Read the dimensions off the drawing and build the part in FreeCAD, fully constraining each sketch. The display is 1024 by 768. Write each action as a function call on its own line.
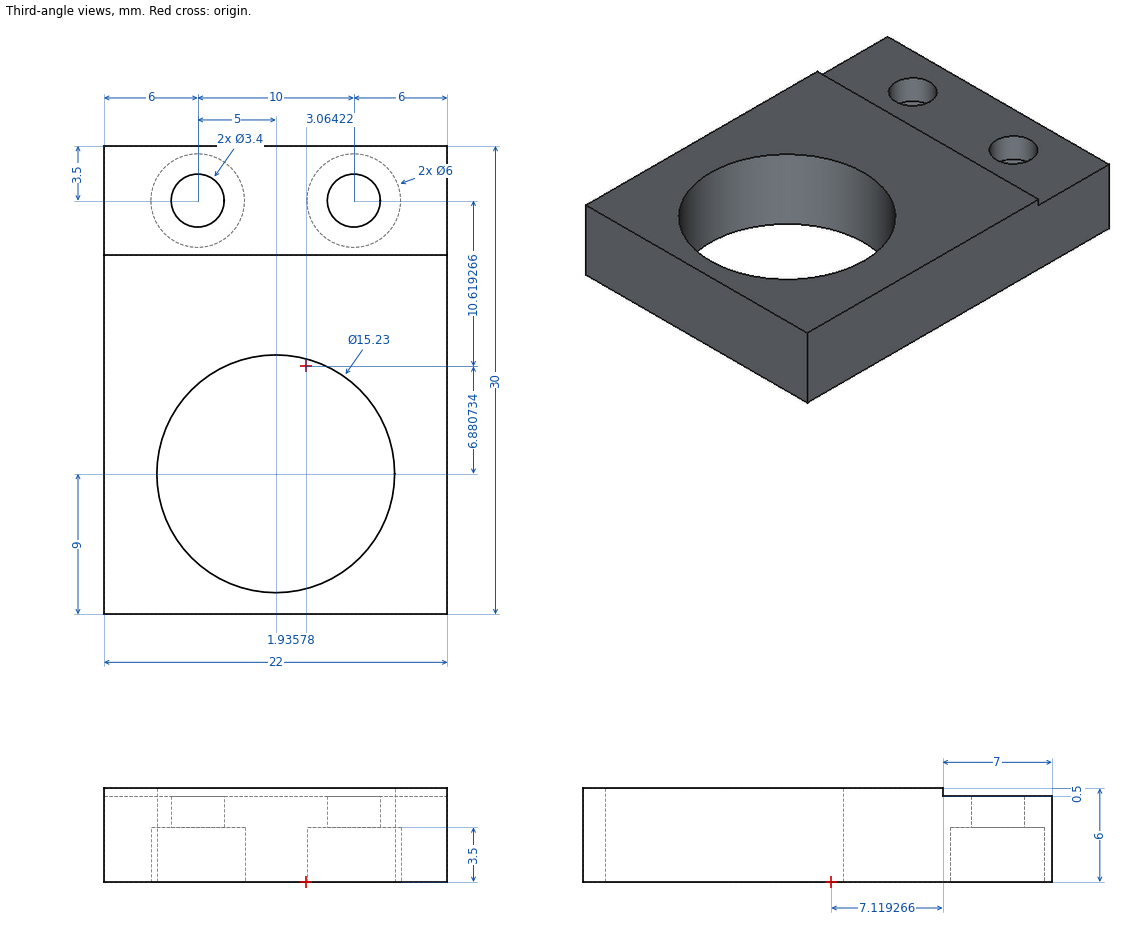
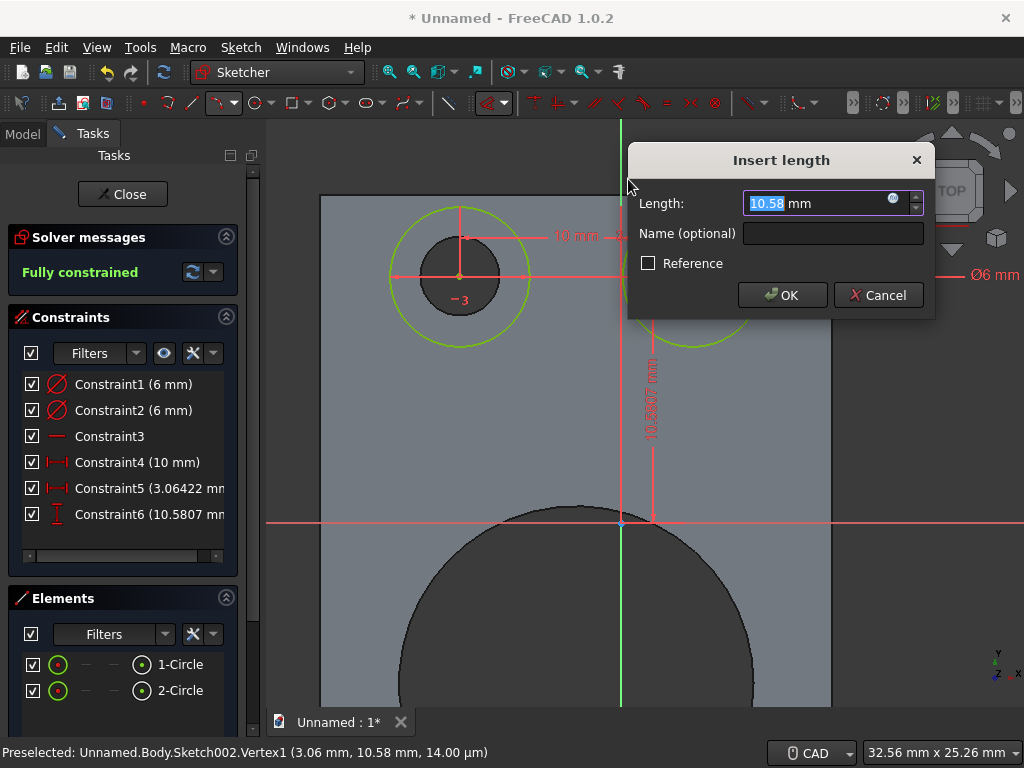
text(10.619266)
key(Return)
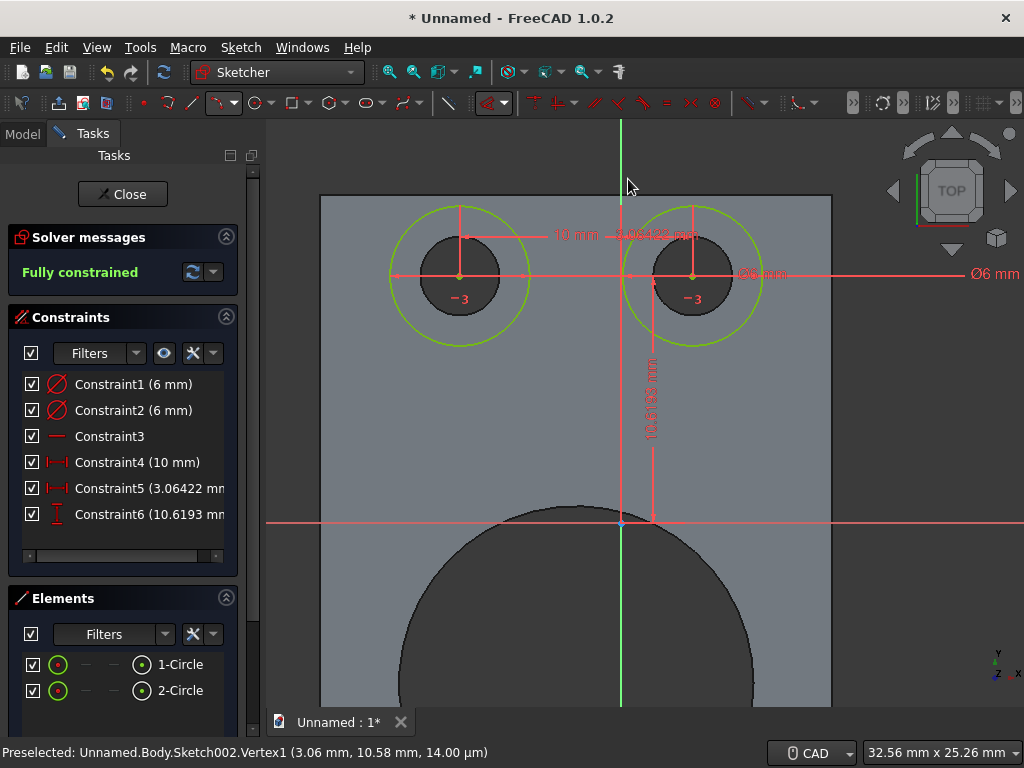
click(123, 194)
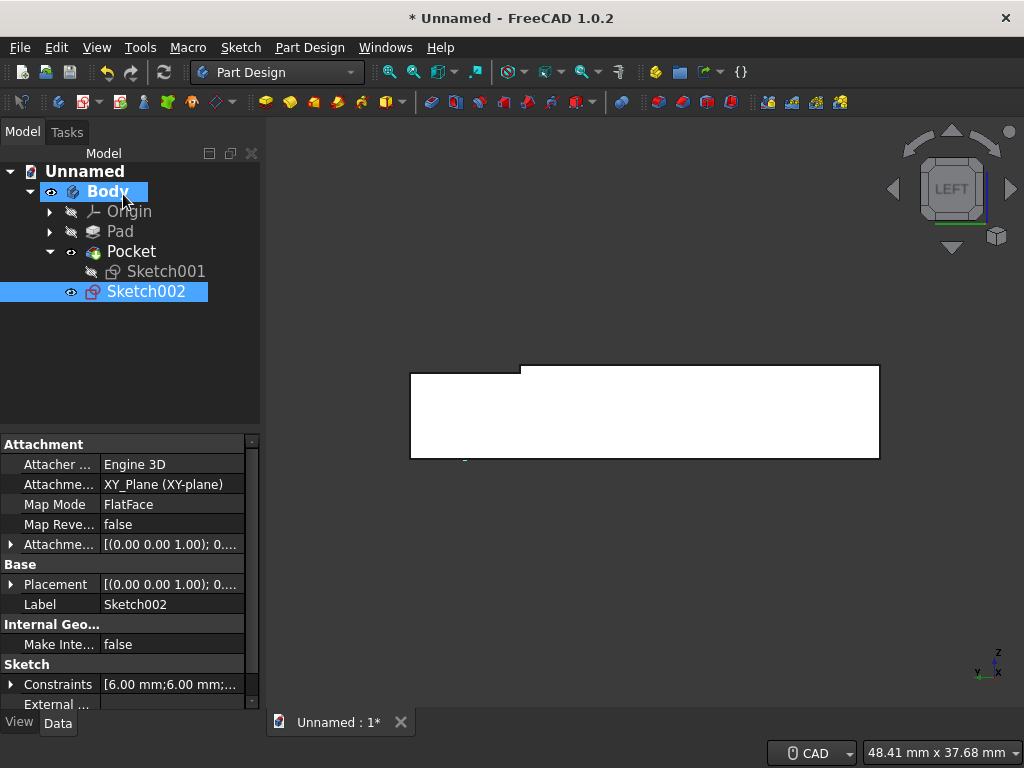
click(432, 102)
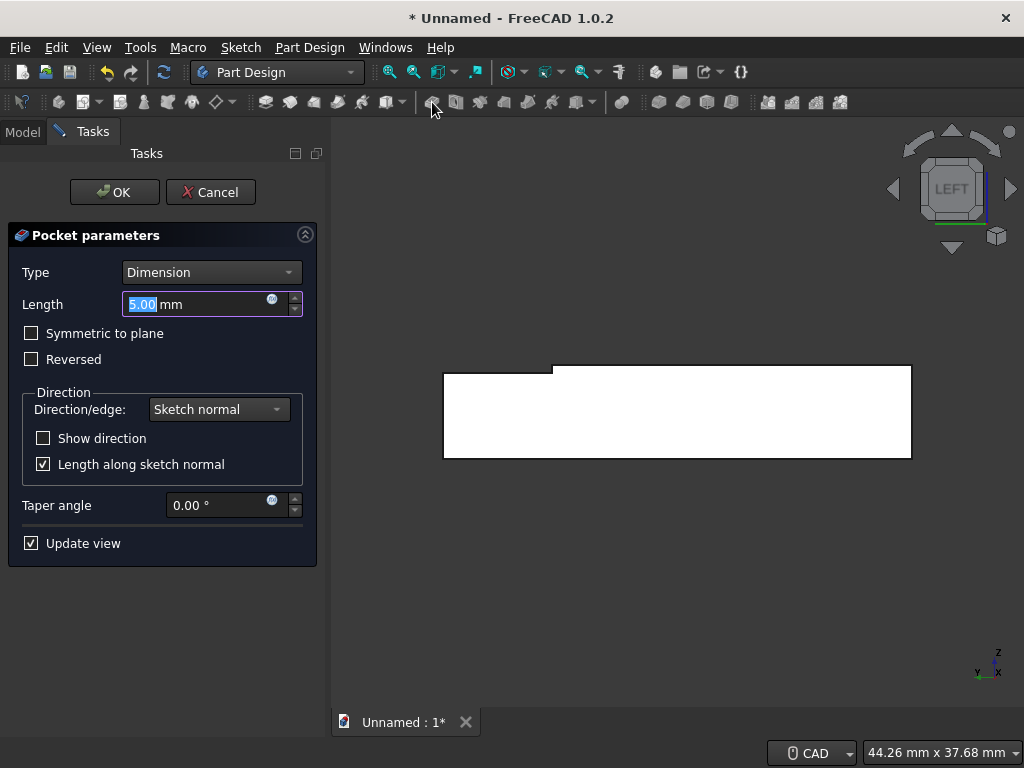
text(3.5)
key(Tab)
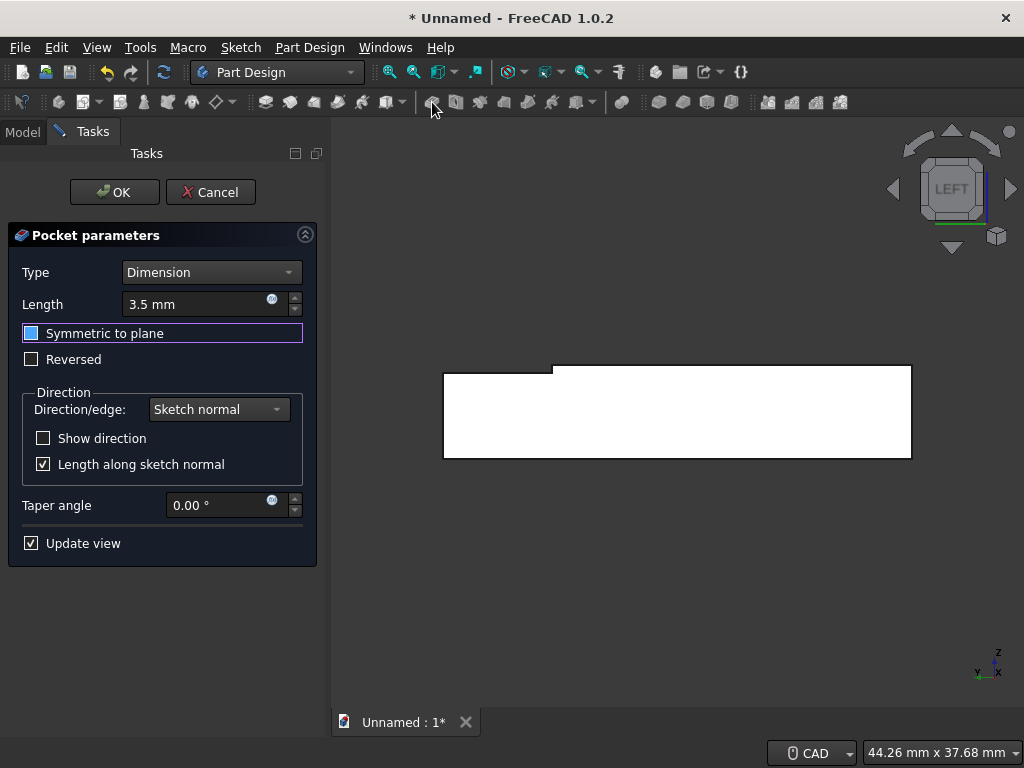
click(30, 359)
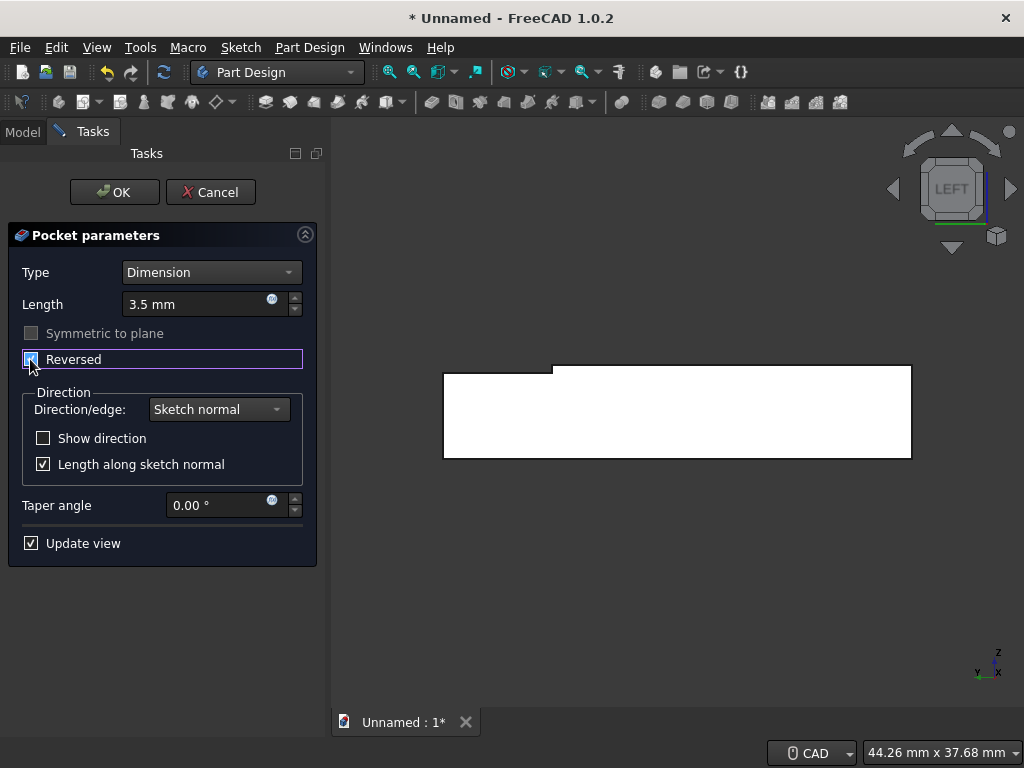
click(115, 192)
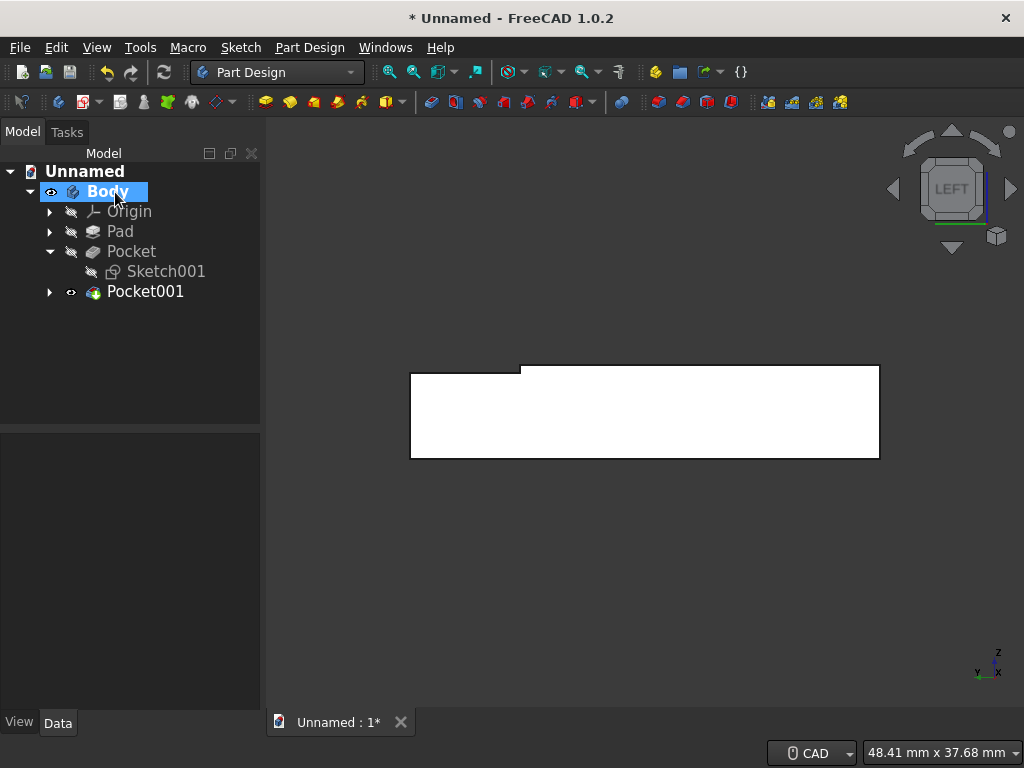
key(0)